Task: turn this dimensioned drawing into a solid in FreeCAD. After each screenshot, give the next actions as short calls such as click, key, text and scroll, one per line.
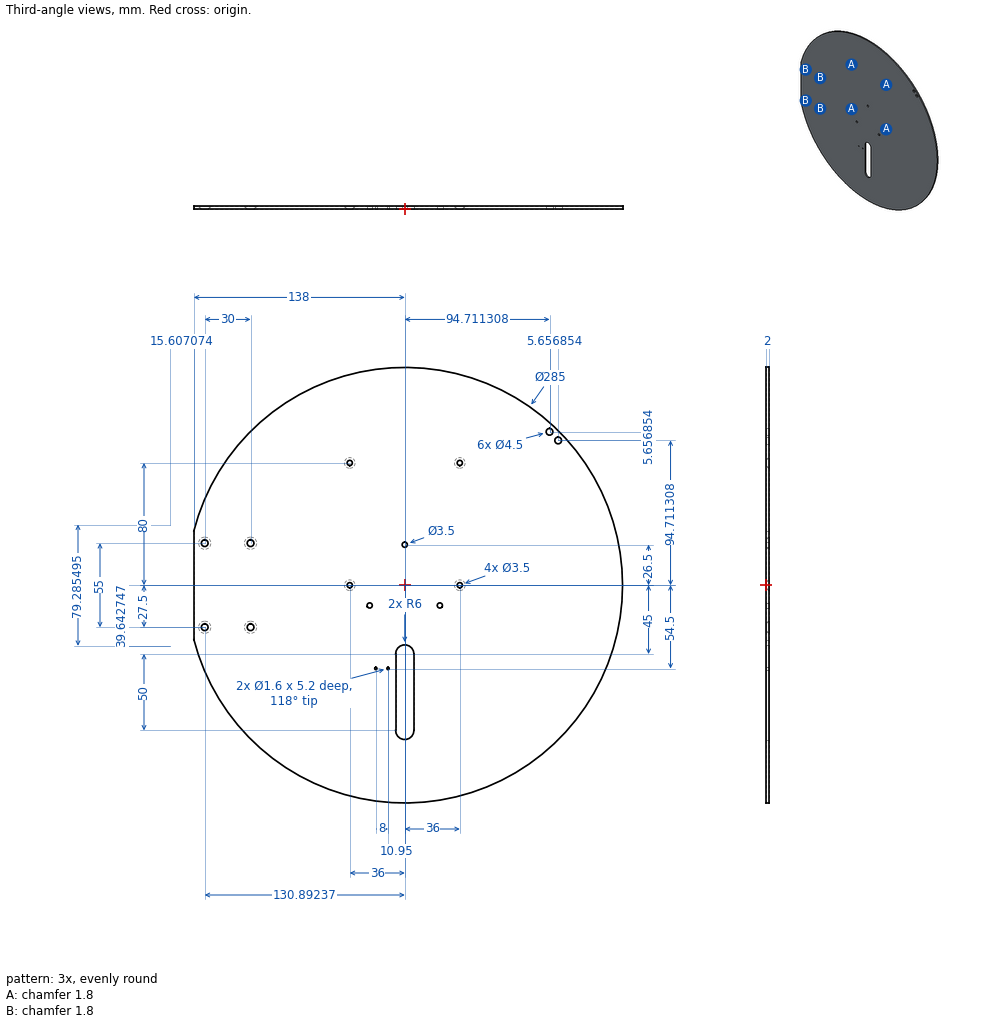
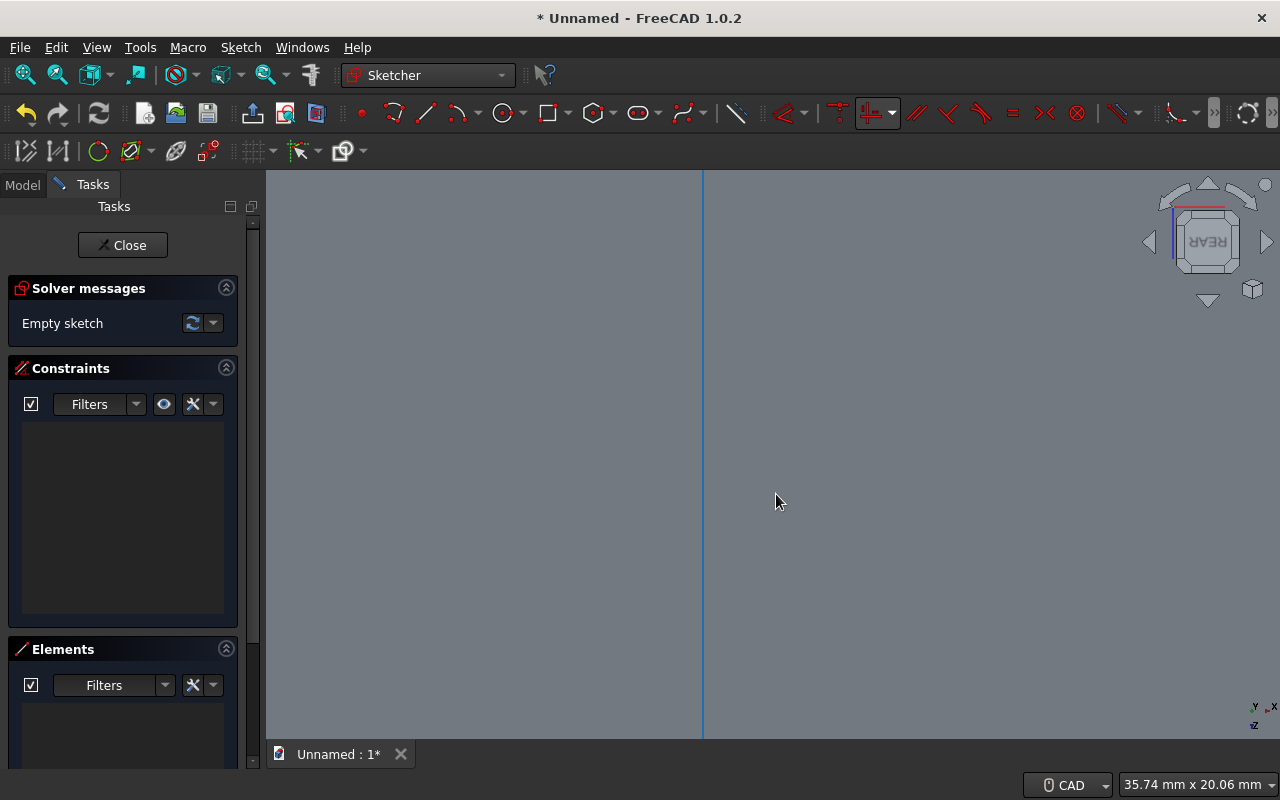
scroll(703, 436, up, 6)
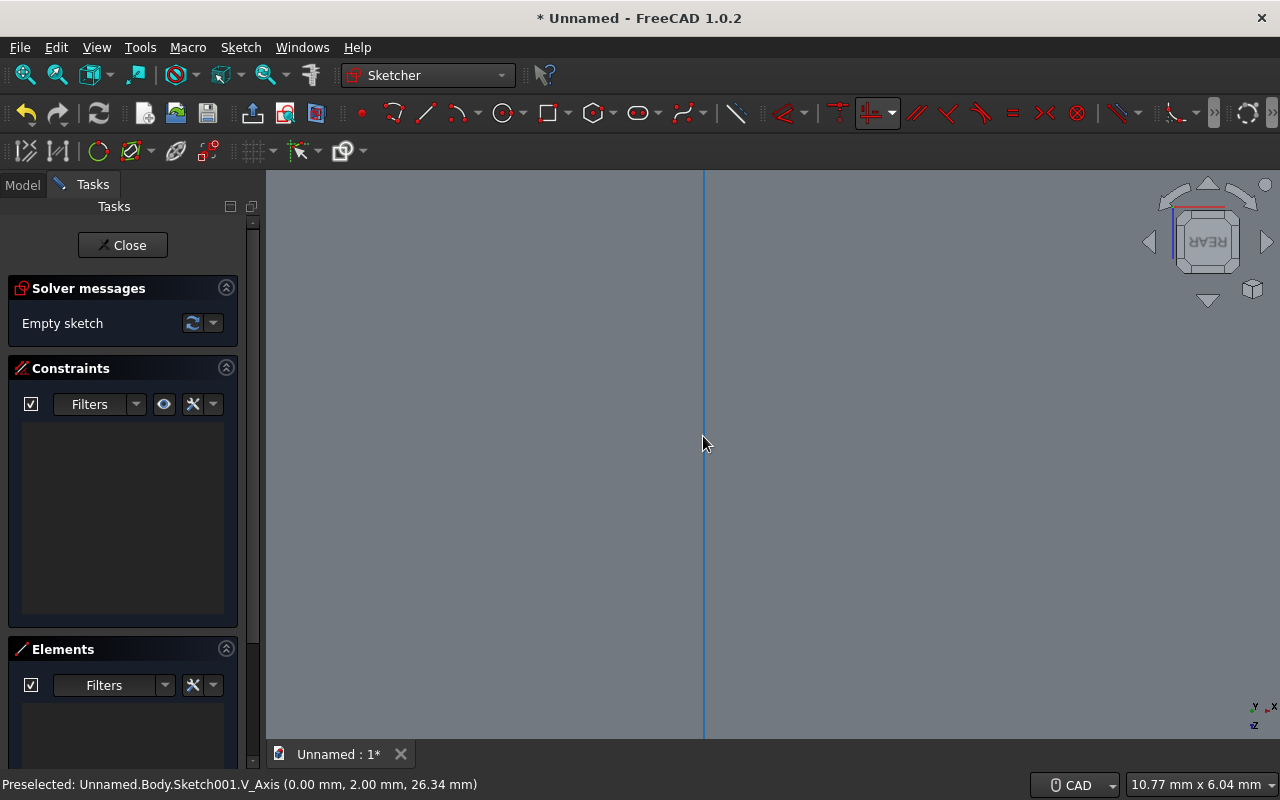
click(504, 114)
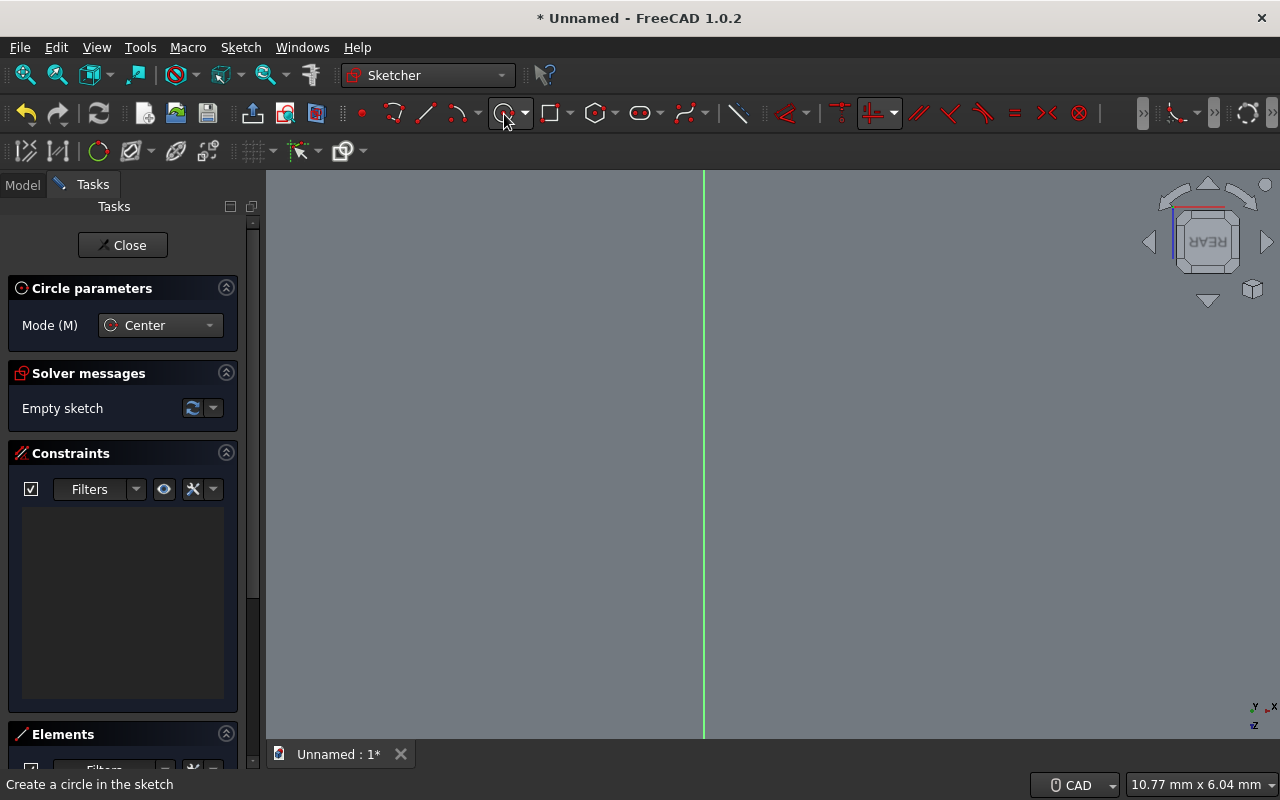
click(704, 453)
click(820, 337)
key(Escape)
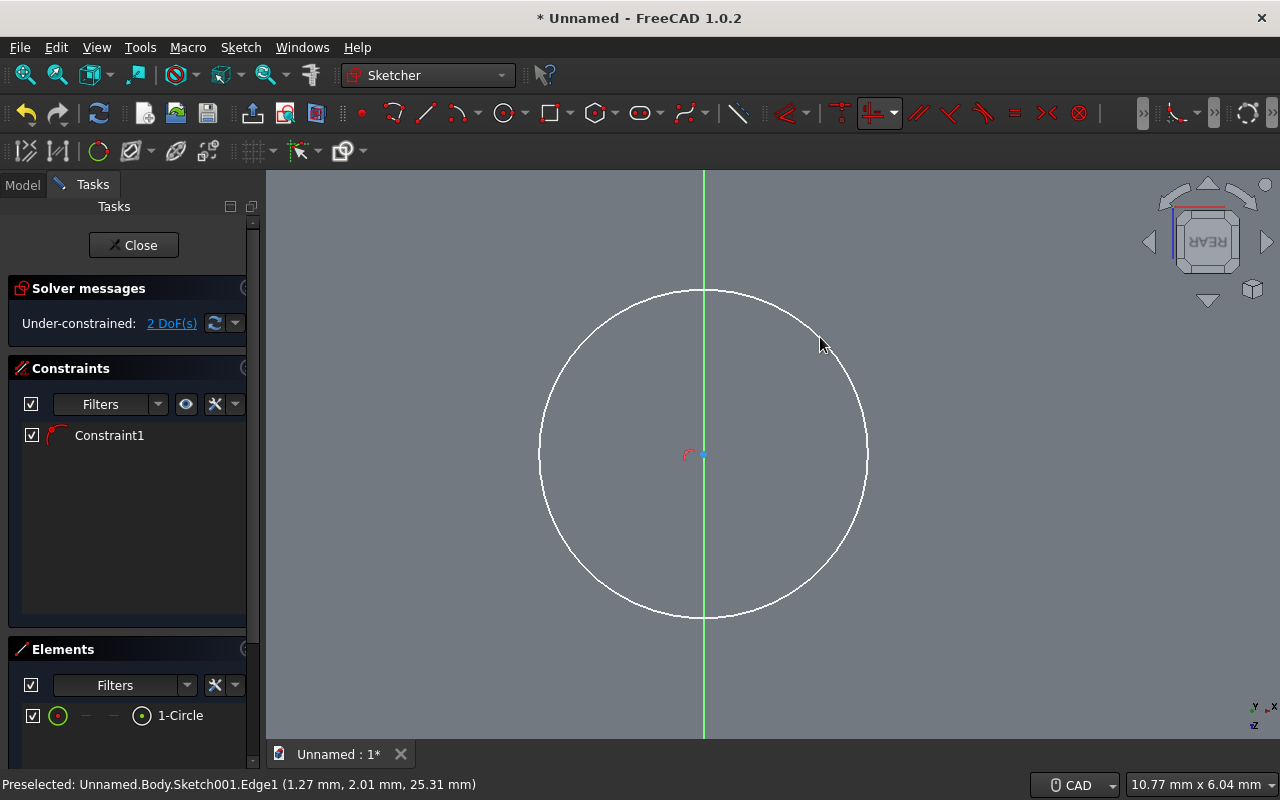
click(786, 114)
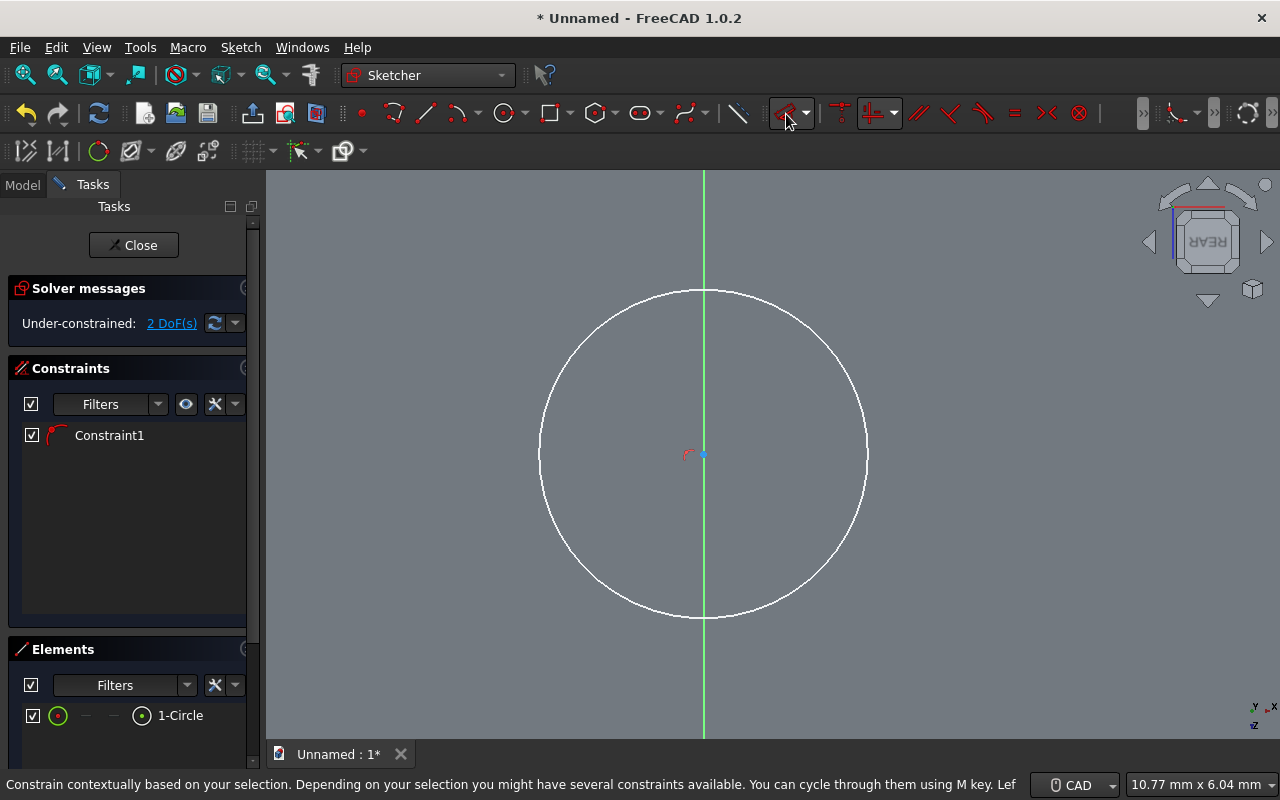
click(819, 337)
click(841, 314)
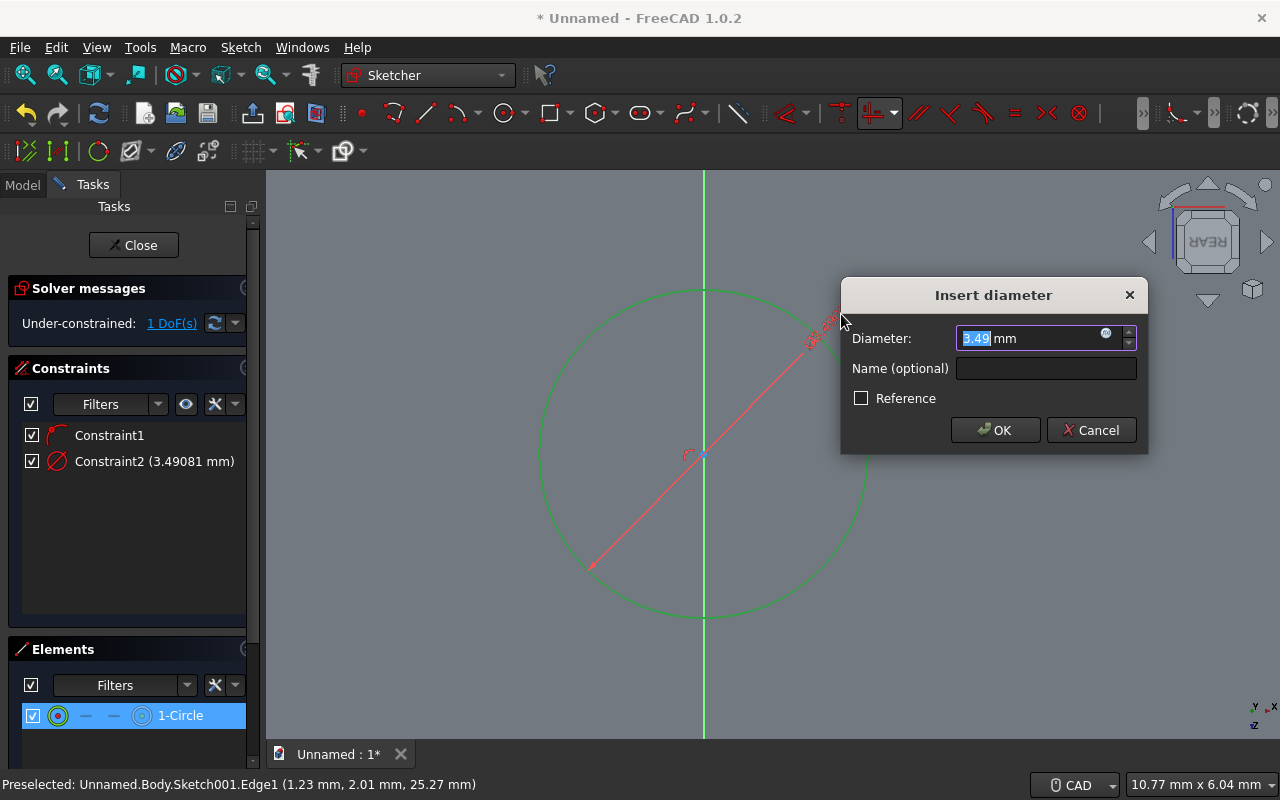
text(3.5)
key(Return)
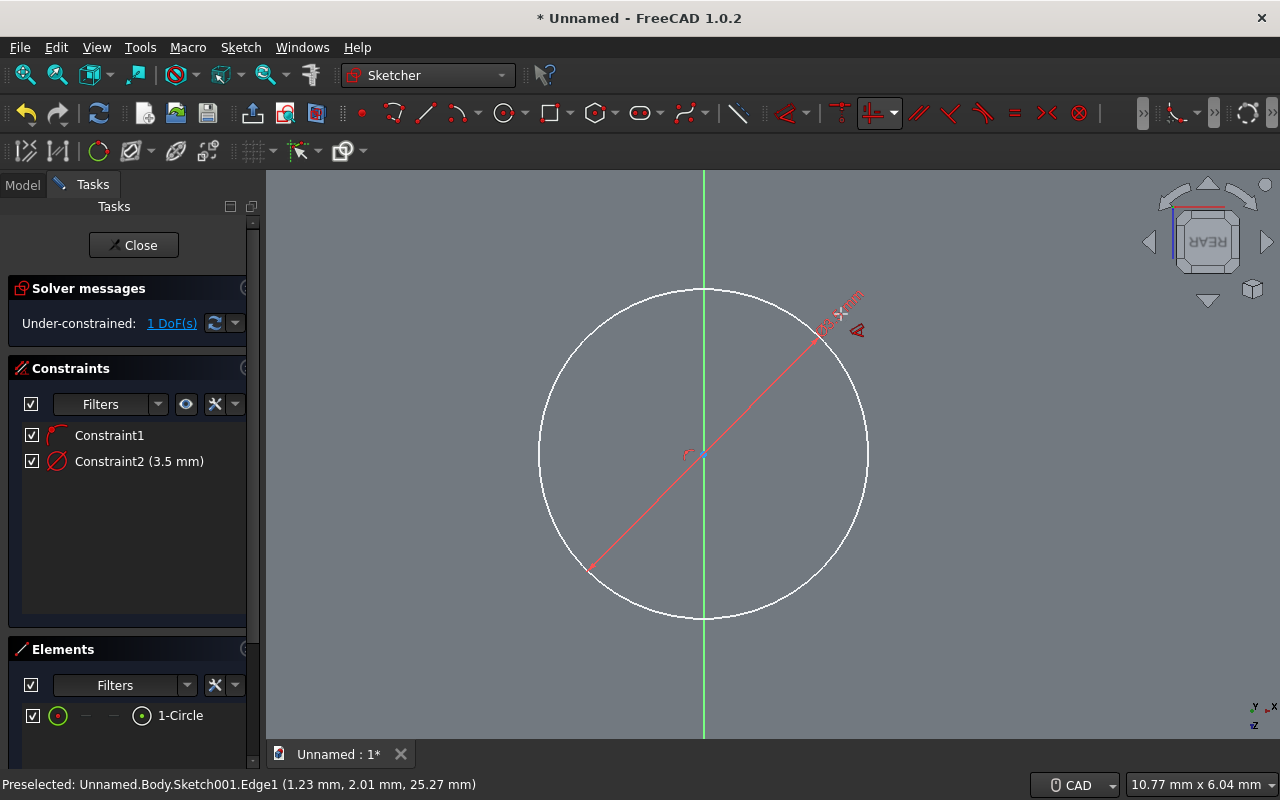
click(704, 454)
click(738, 326)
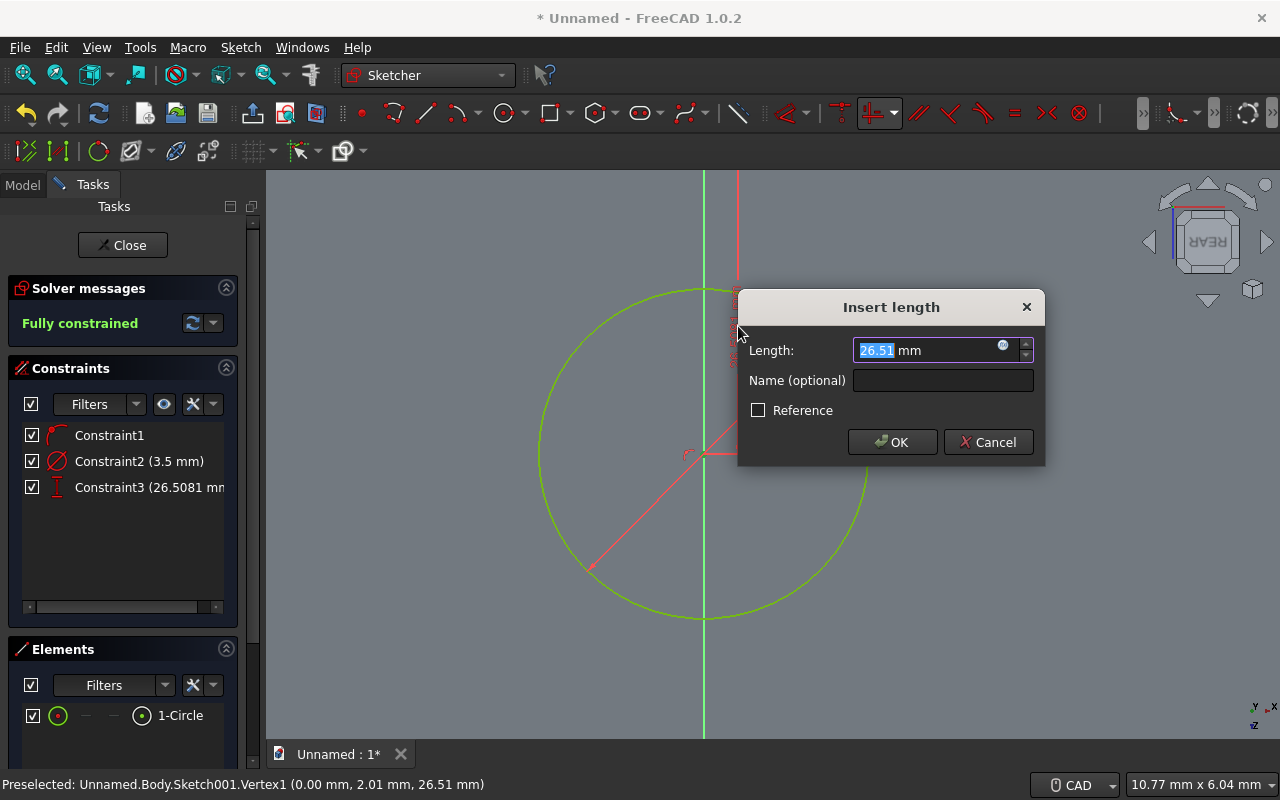
text(26.5)
key(Return)
key(Escape)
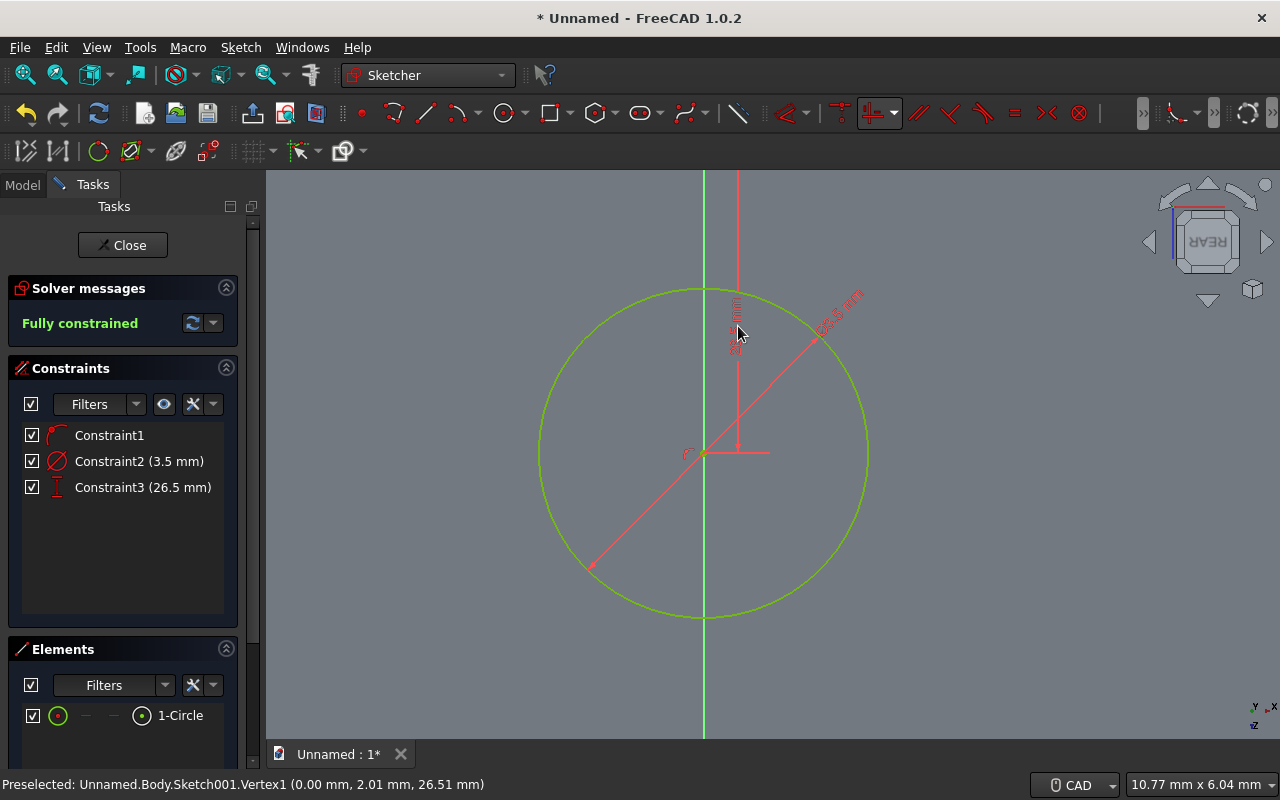
click(123, 245)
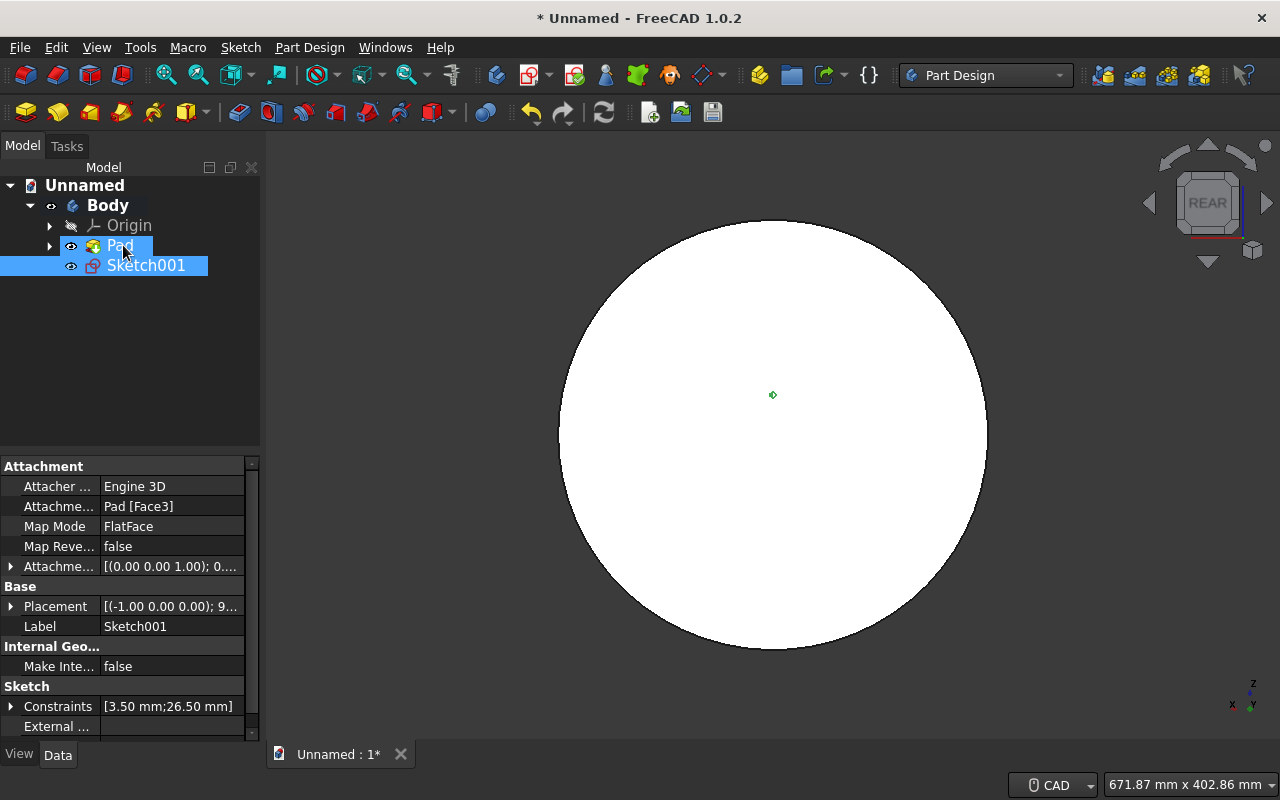
click(240, 112)